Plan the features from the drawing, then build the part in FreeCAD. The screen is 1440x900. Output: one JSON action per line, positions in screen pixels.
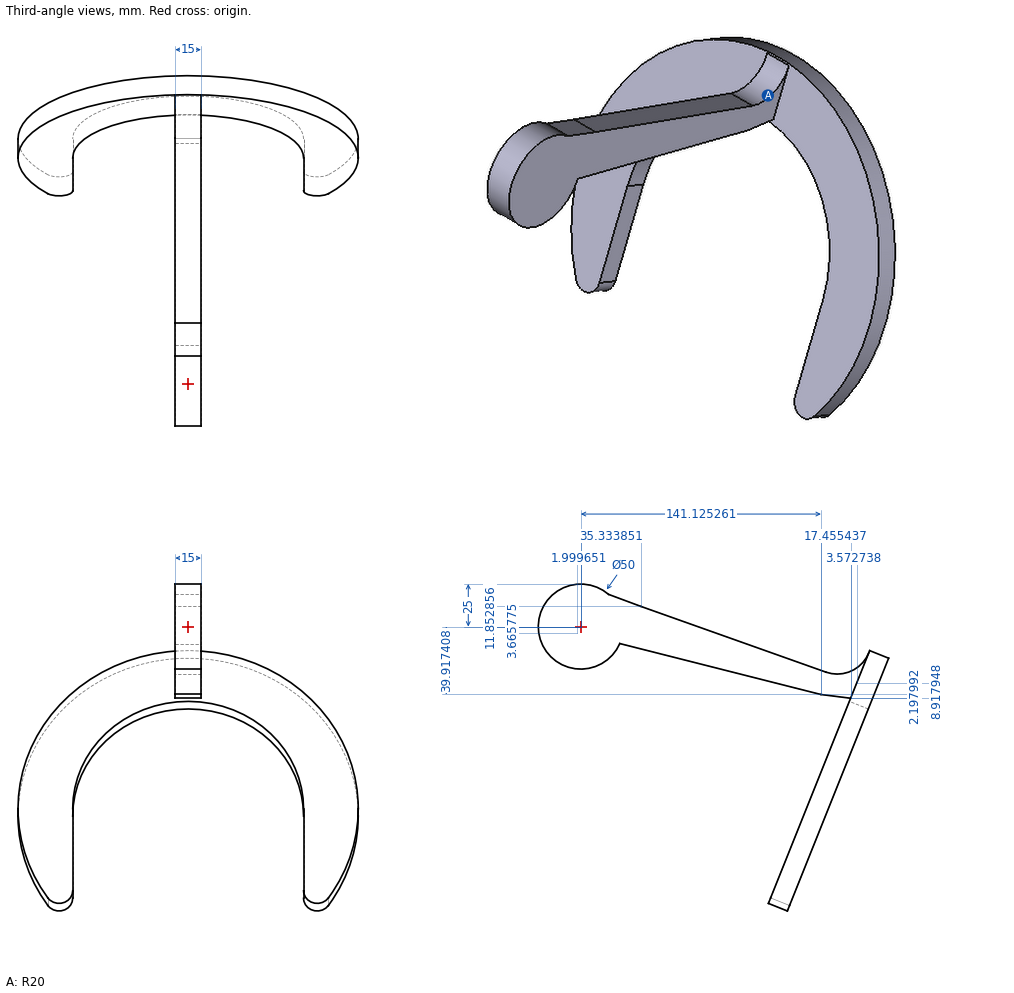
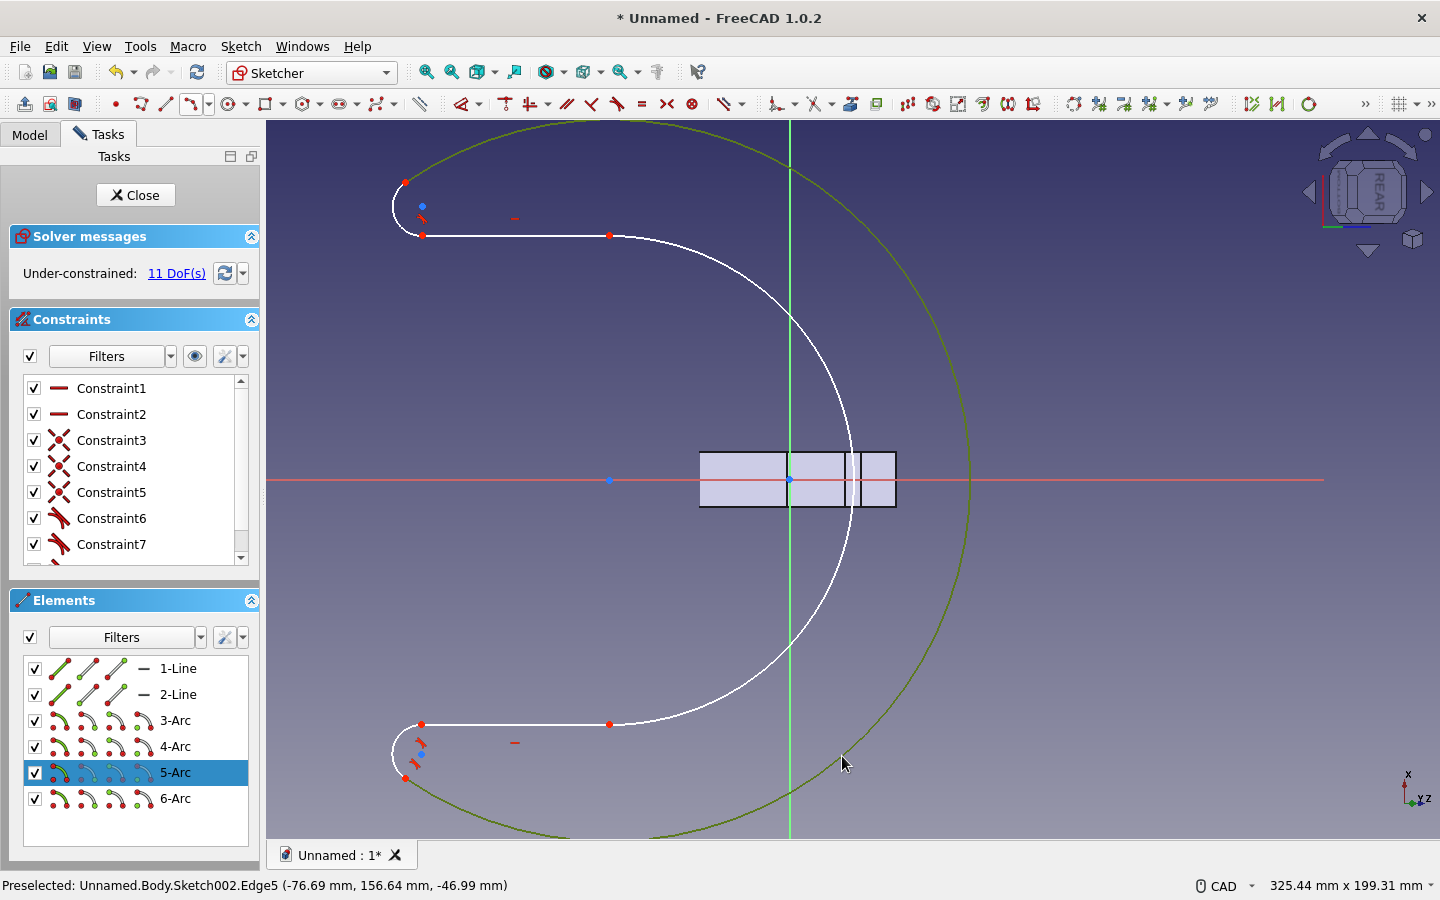
{"action": "left_click", "coordinate": [393, 201]}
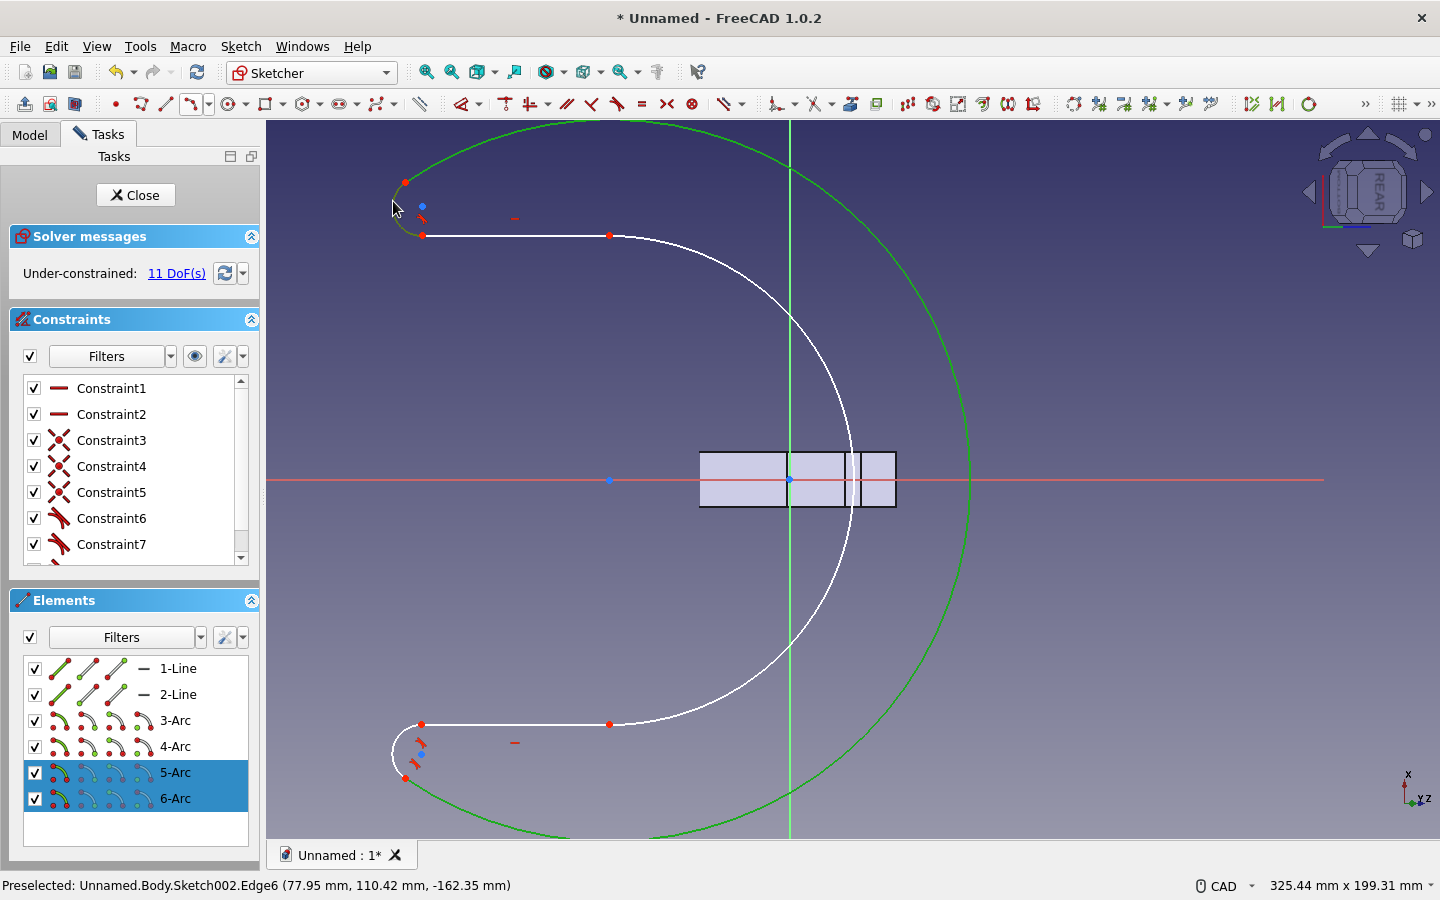
{"action": "left_click", "coordinate": [617, 104]}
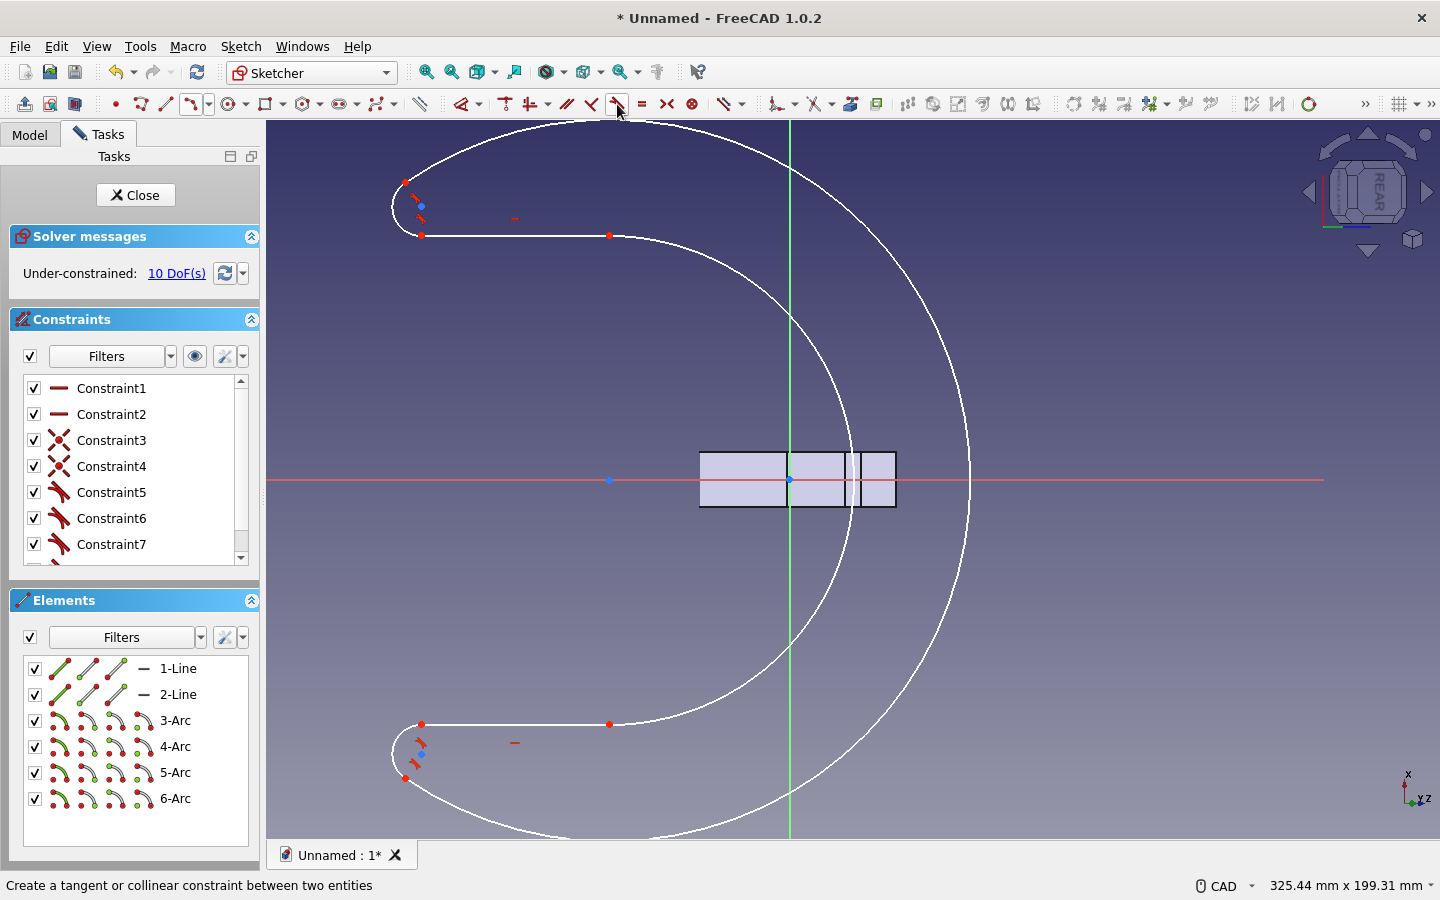
{"action": "left_click", "coordinate": [807, 624]}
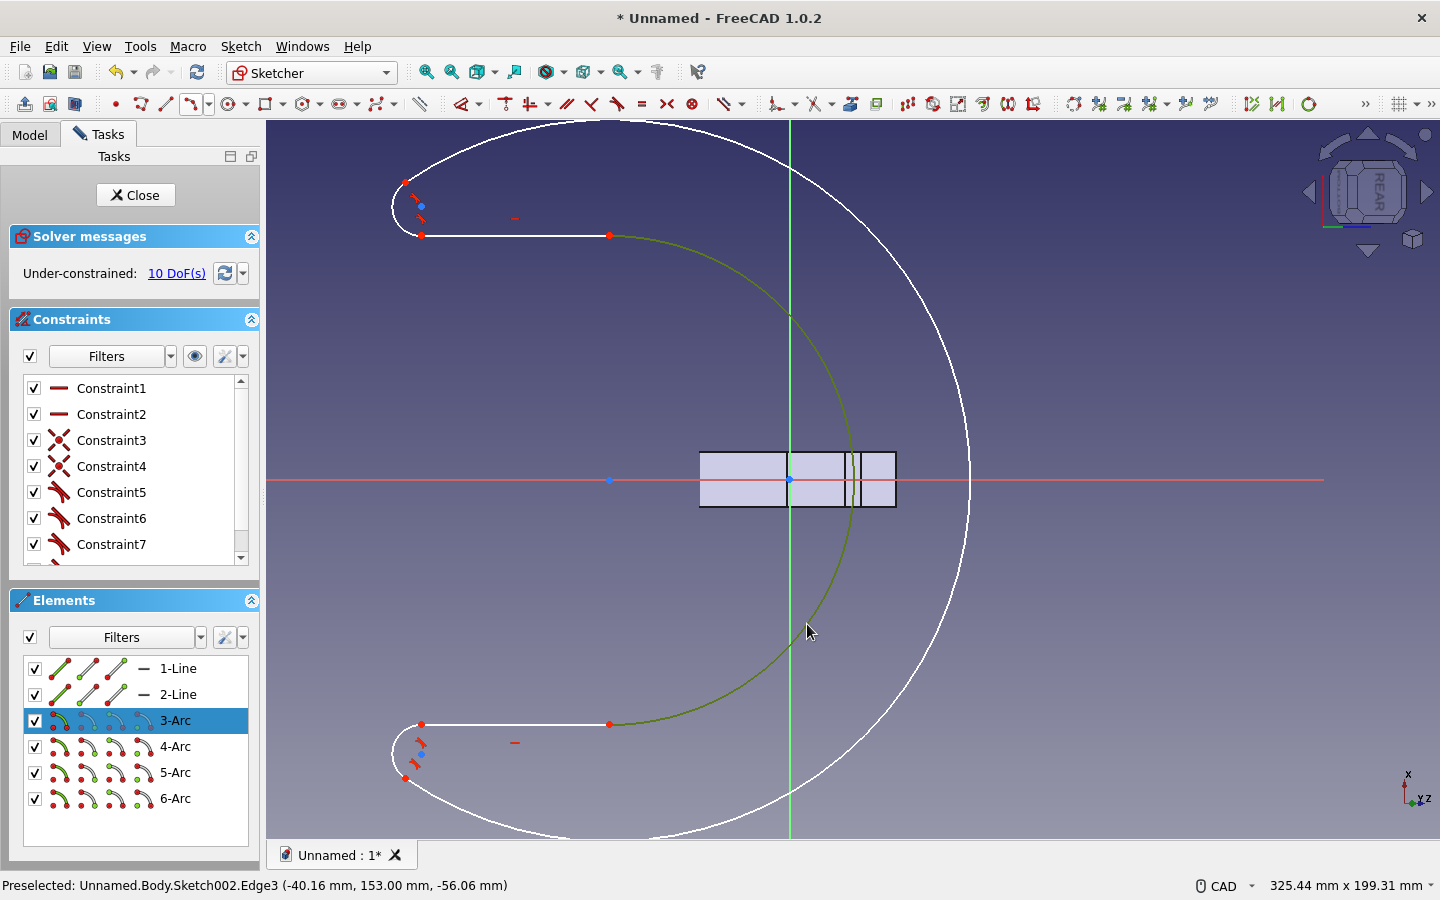
{"action": "left_click", "coordinate": [842, 756]}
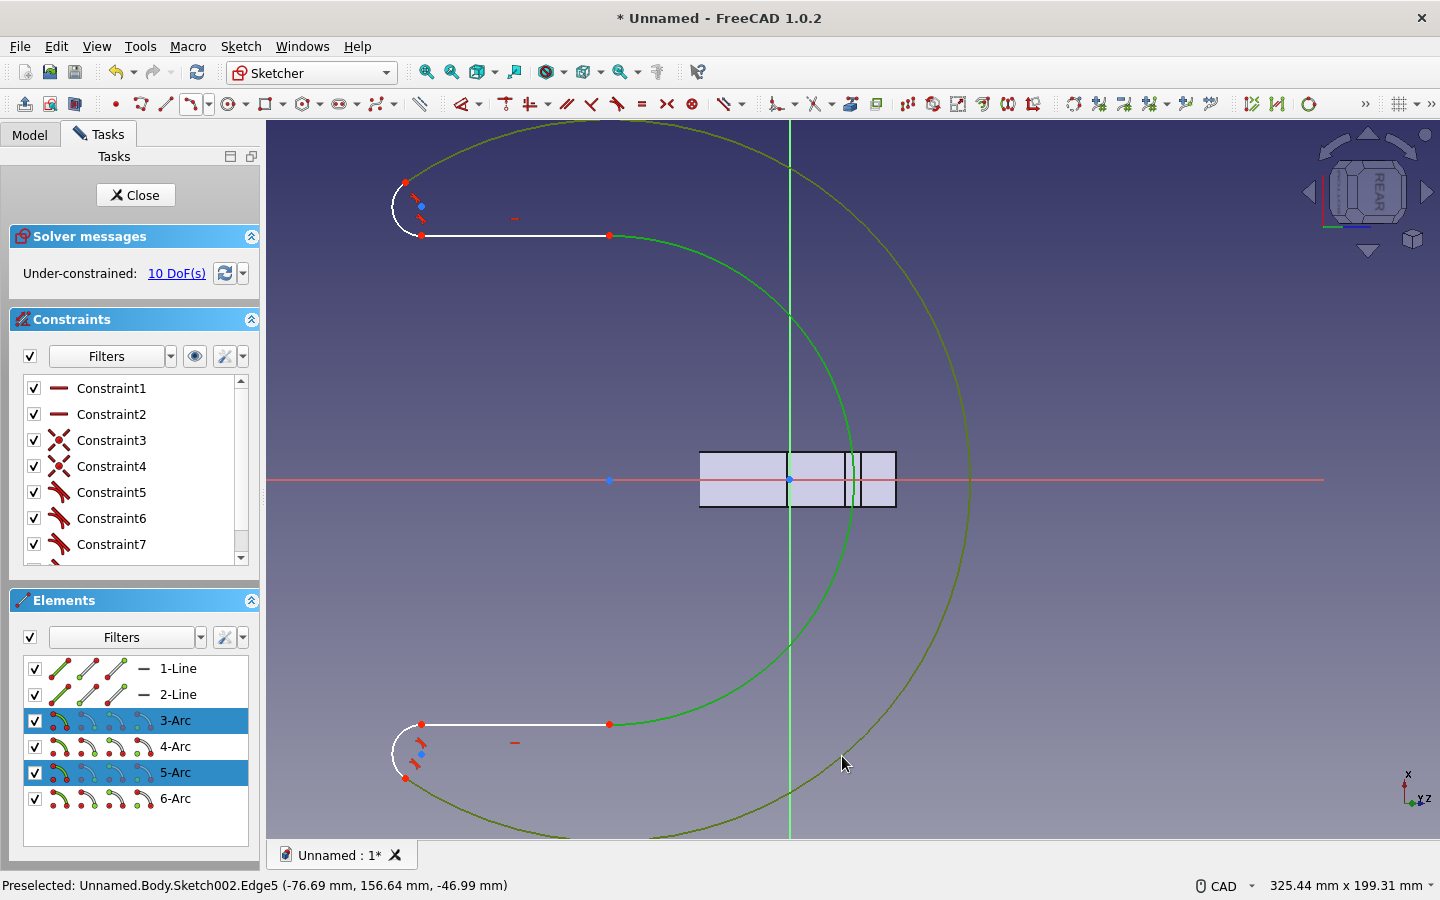
{"action": "left_click", "coordinate": [505, 104]}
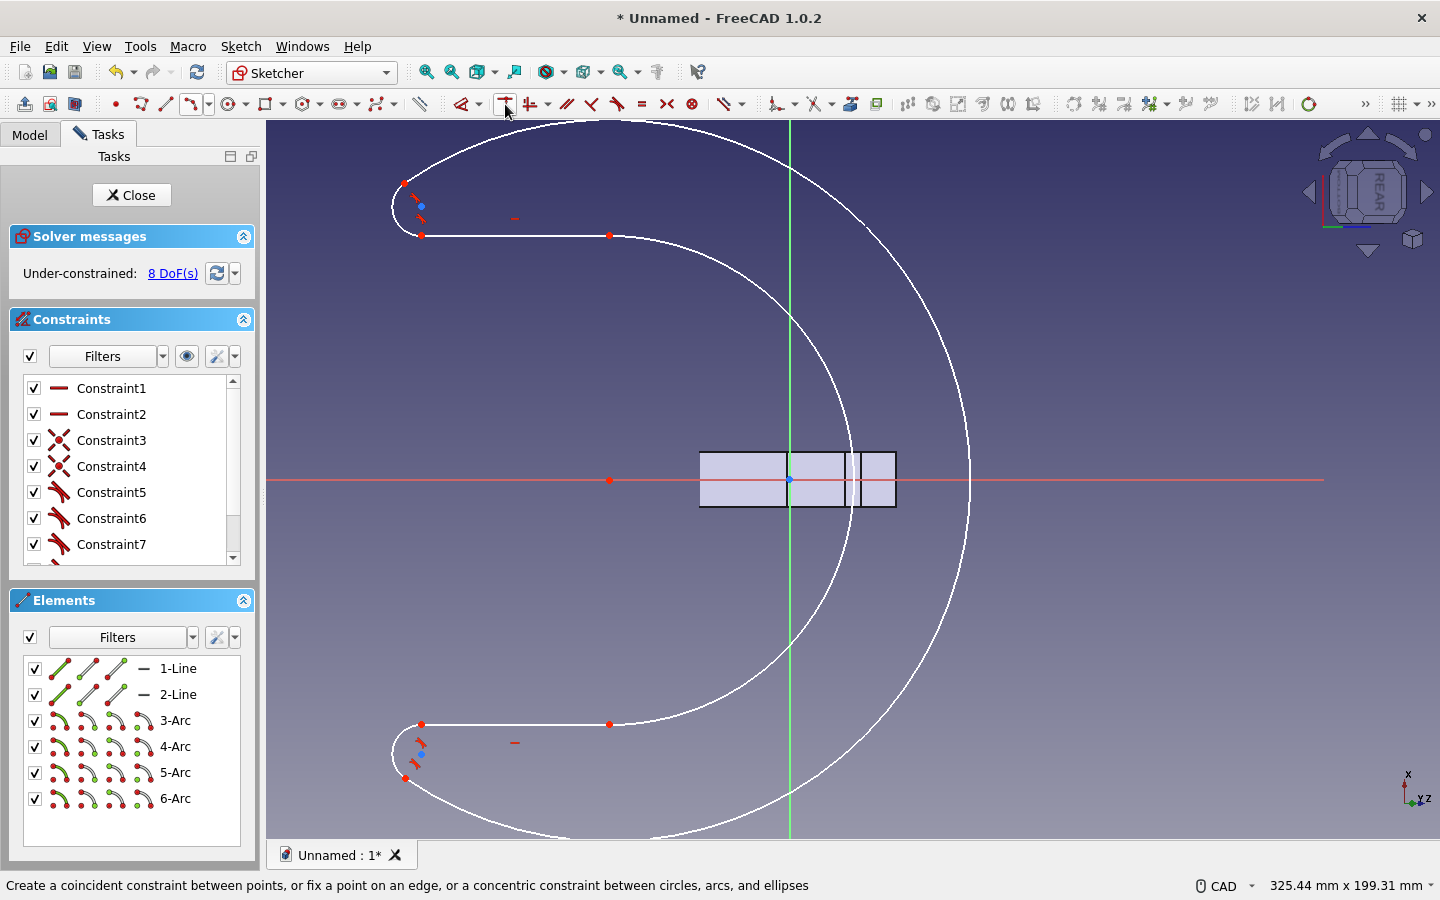
{"action": "left_click", "coordinate": [401, 733]}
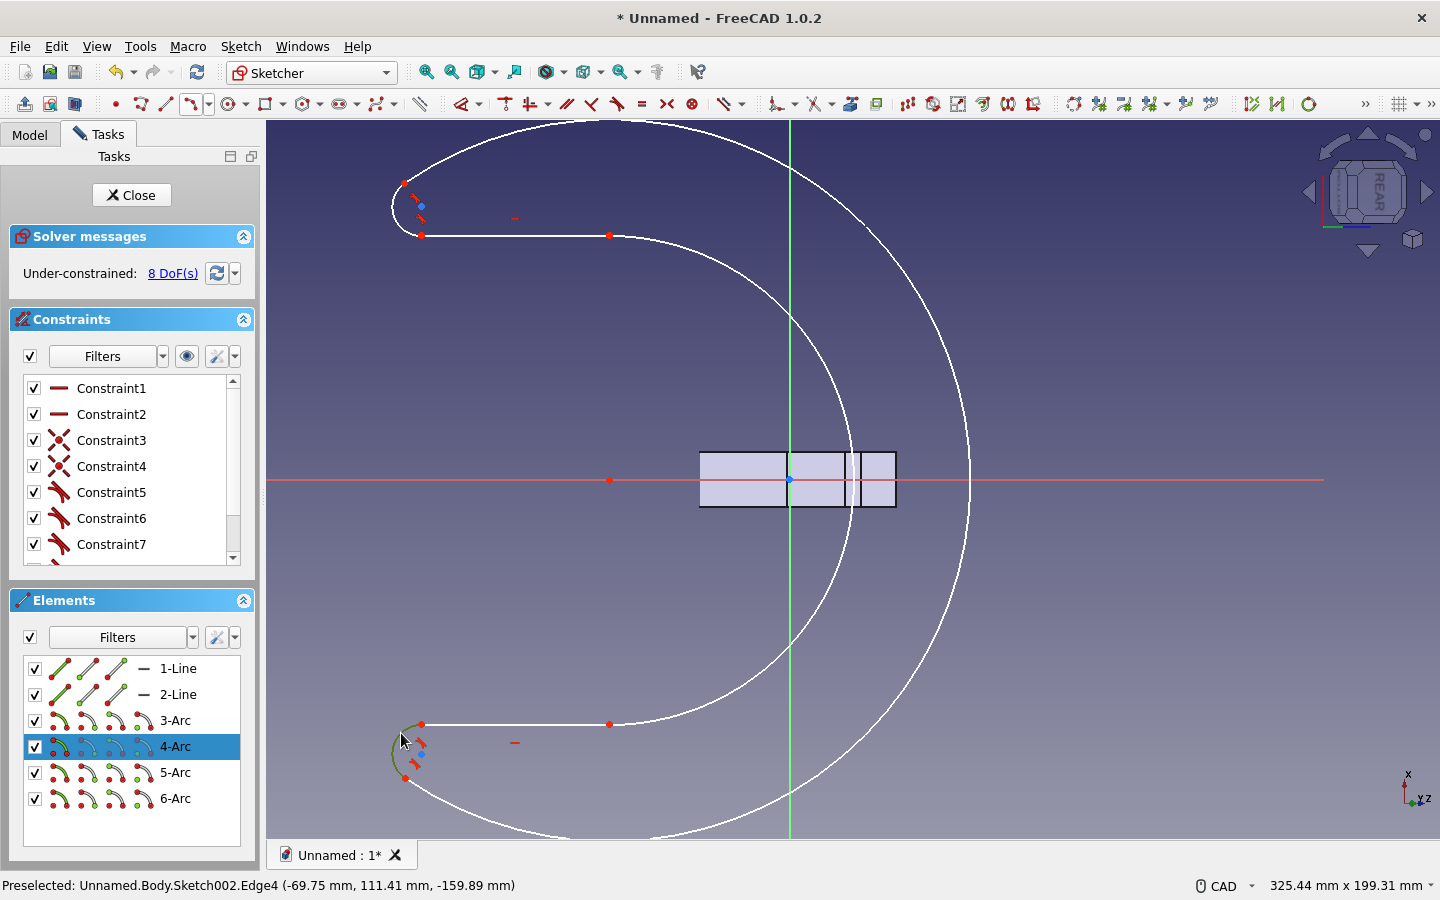
{"action": "left_click", "coordinate": [393, 201]}